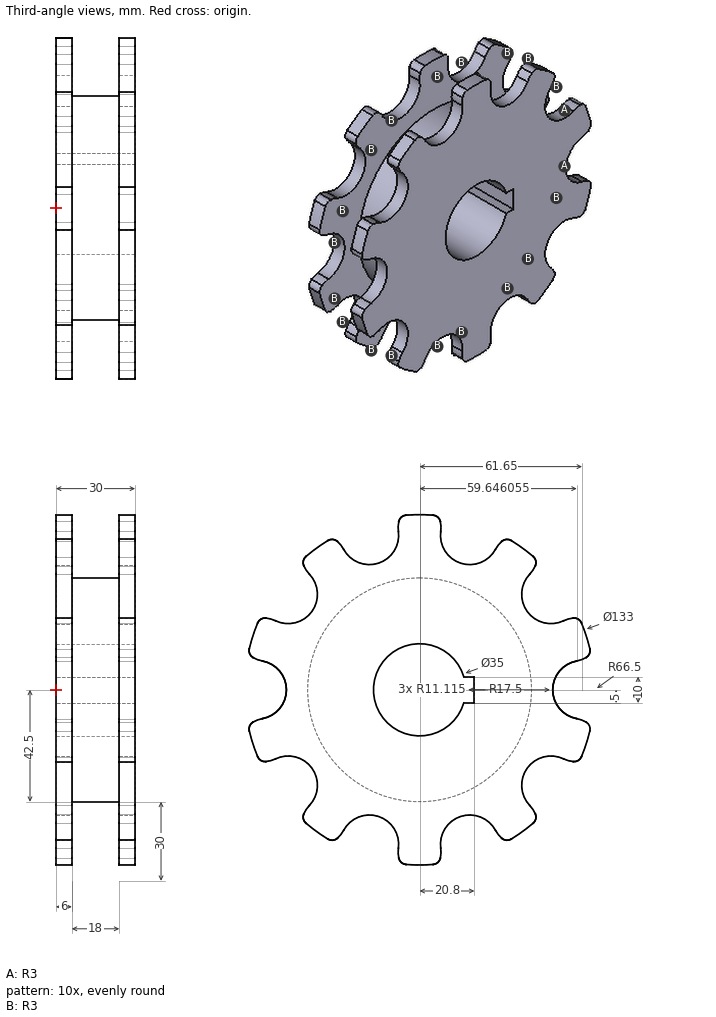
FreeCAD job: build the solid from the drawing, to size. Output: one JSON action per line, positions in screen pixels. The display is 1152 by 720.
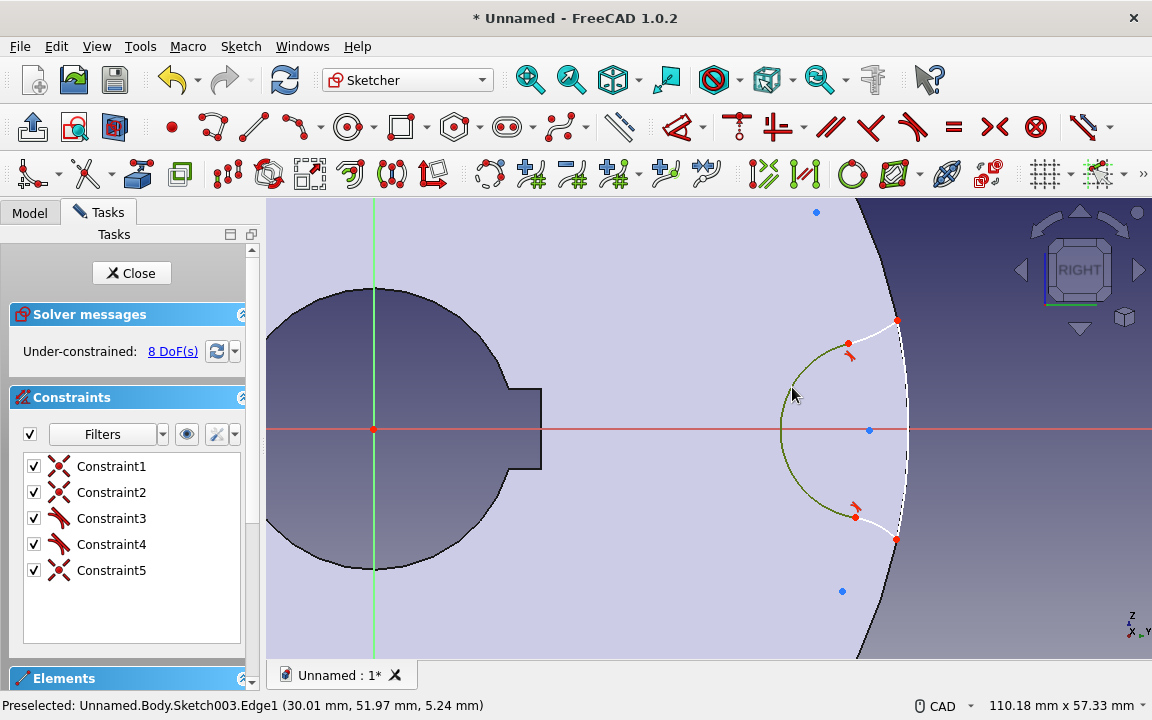
{"action": "left_click", "coordinate": [886, 530]}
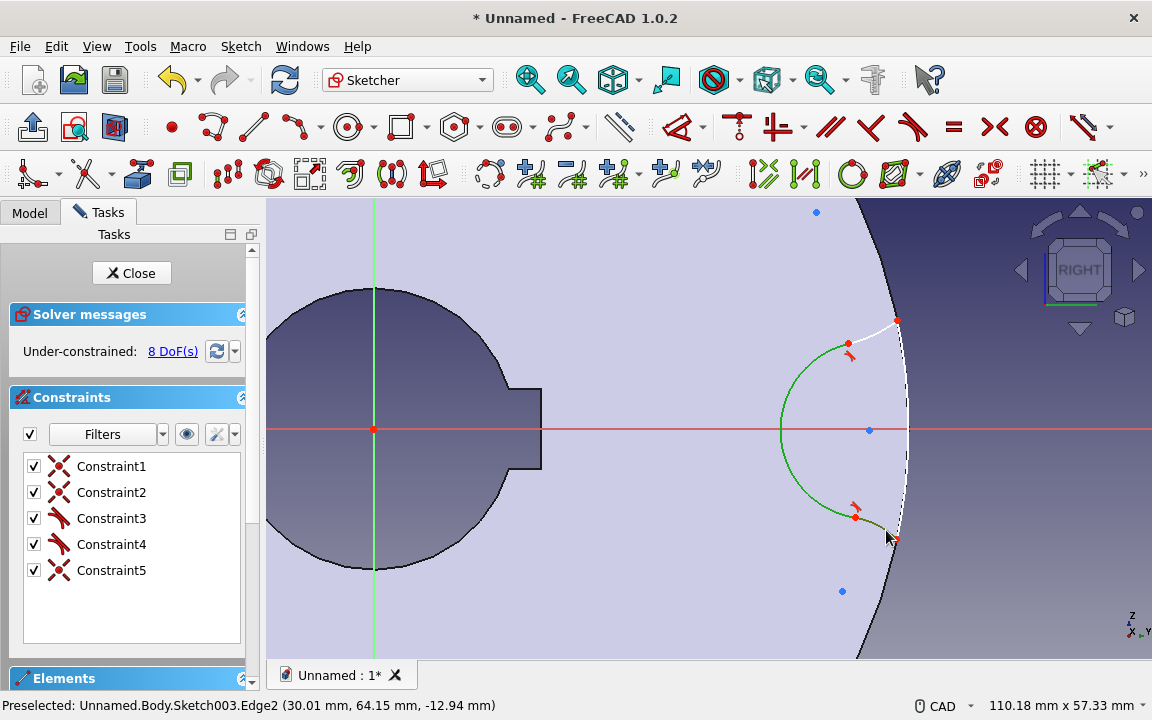
{"action": "left_click", "coordinate": [864, 339]}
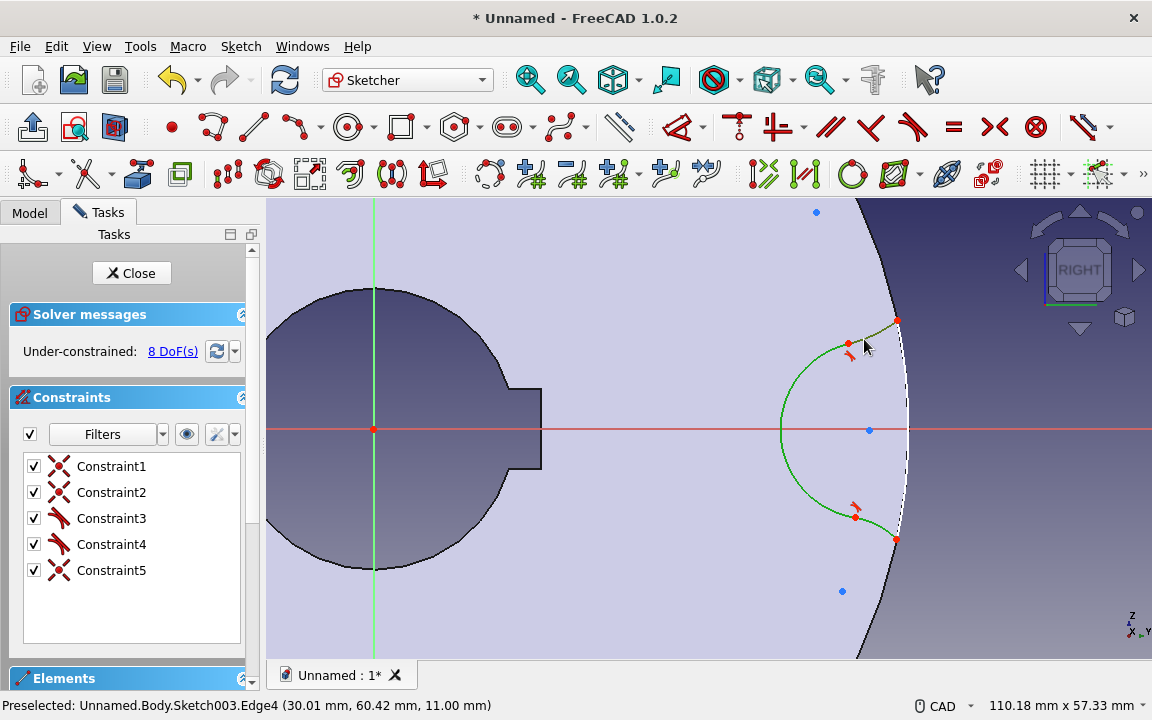
{"action": "left_click", "coordinate": [954, 128]}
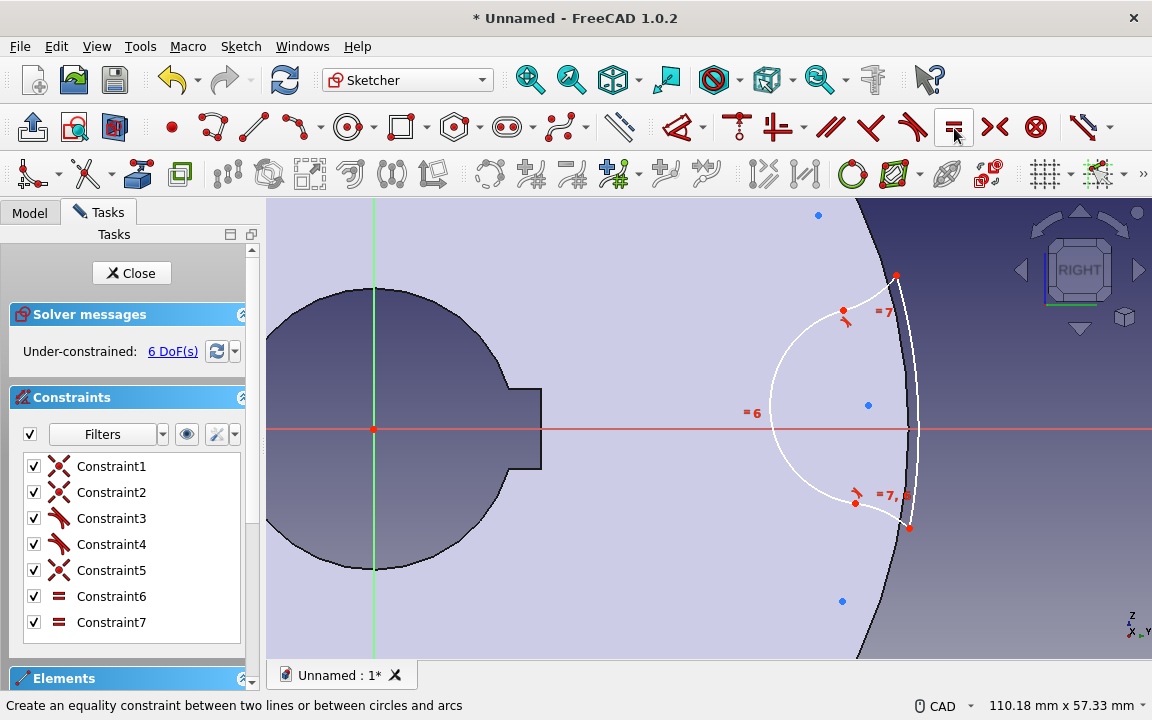
{"action": "left_click", "coordinate": [869, 406]}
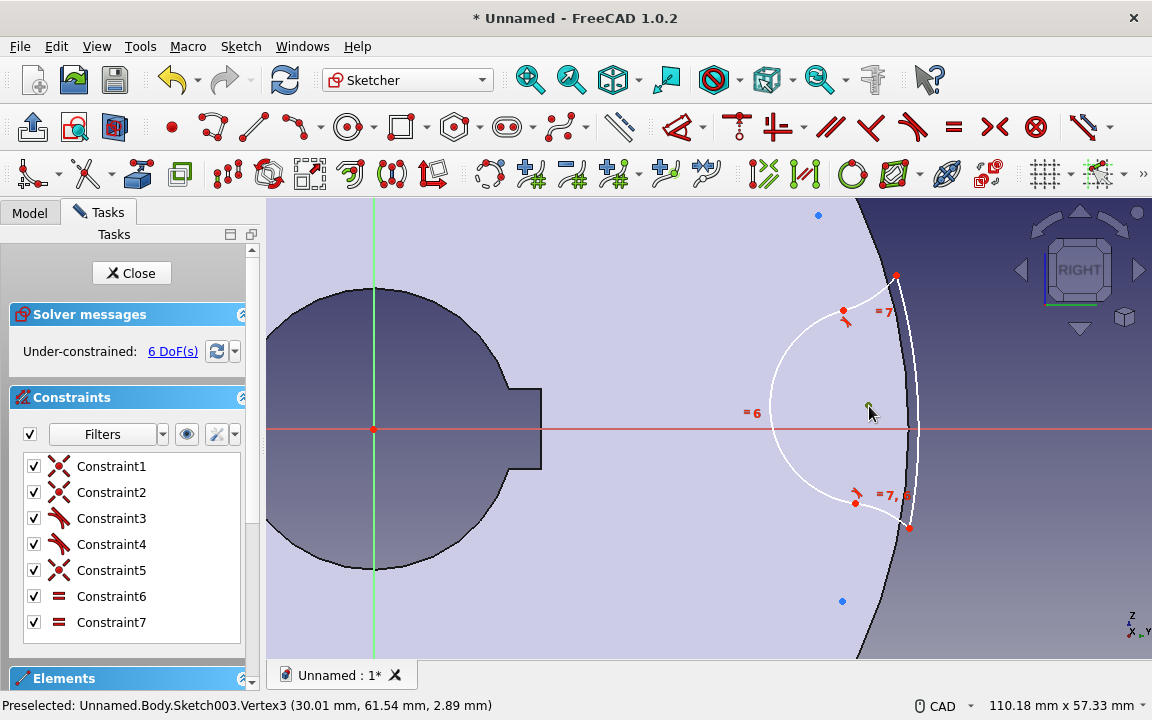
{"action": "left_click", "coordinate": [344, 429]}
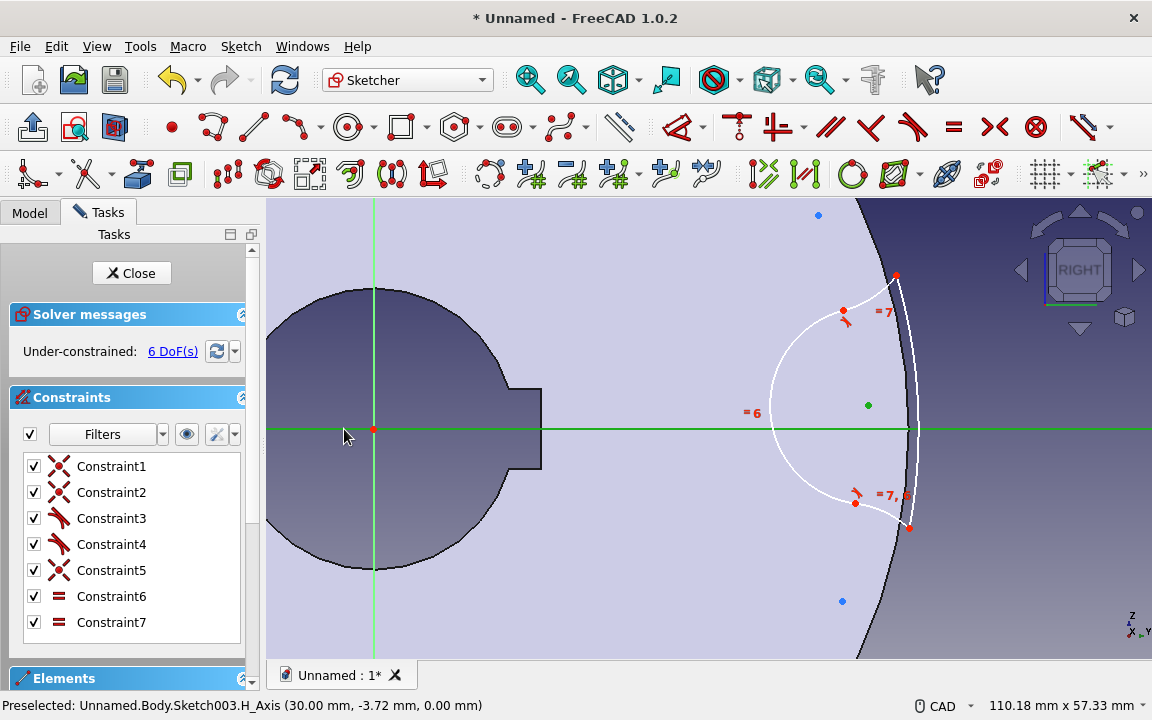
{"action": "left_click", "coordinate": [737, 128]}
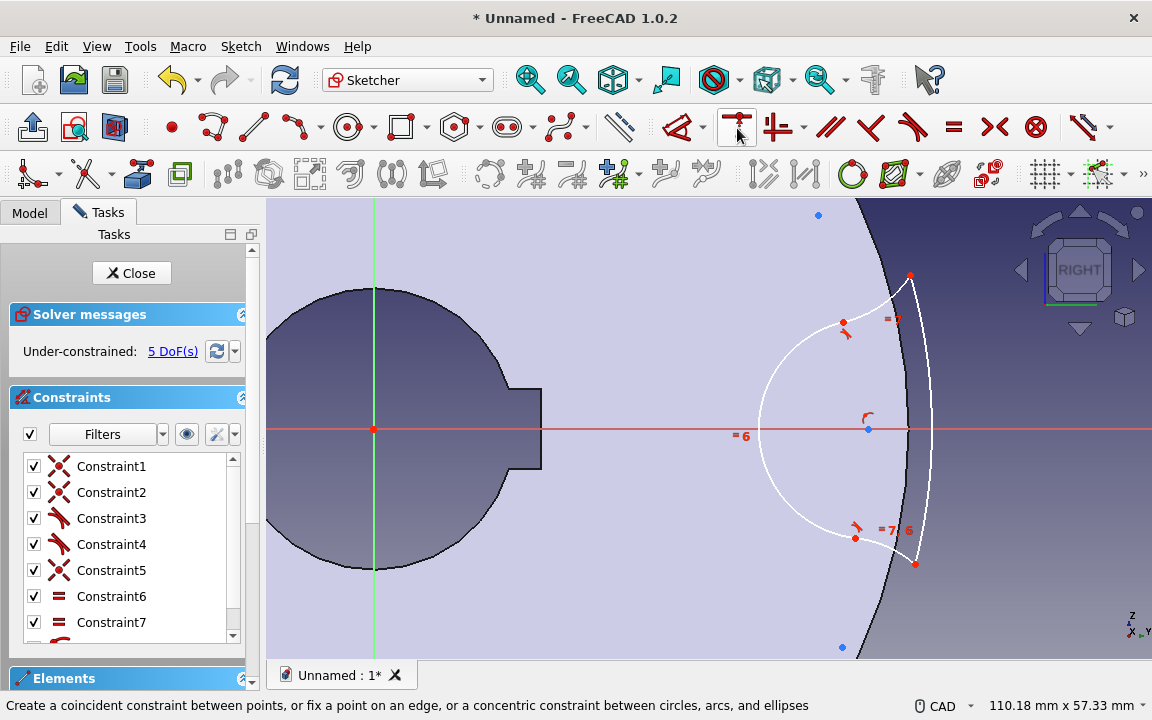
{"action": "left_click", "coordinate": [676, 128]}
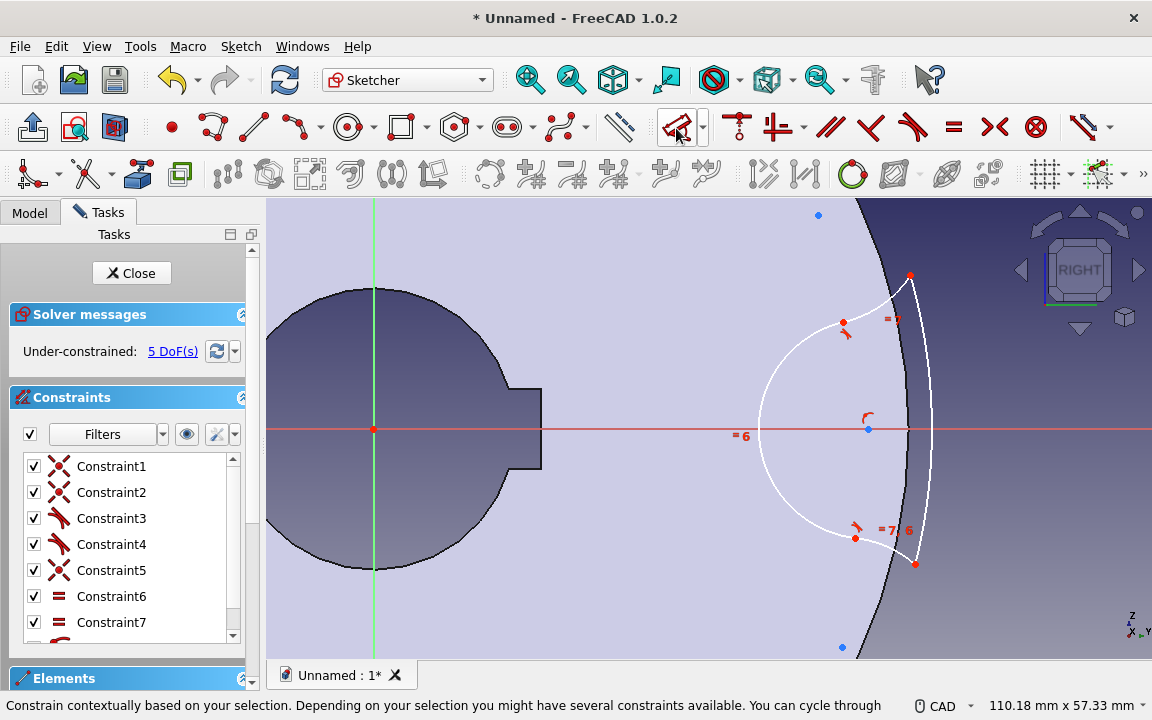
{"action": "left_click", "coordinate": [772, 376]}
{"action": "left_click", "coordinate": [744, 361]}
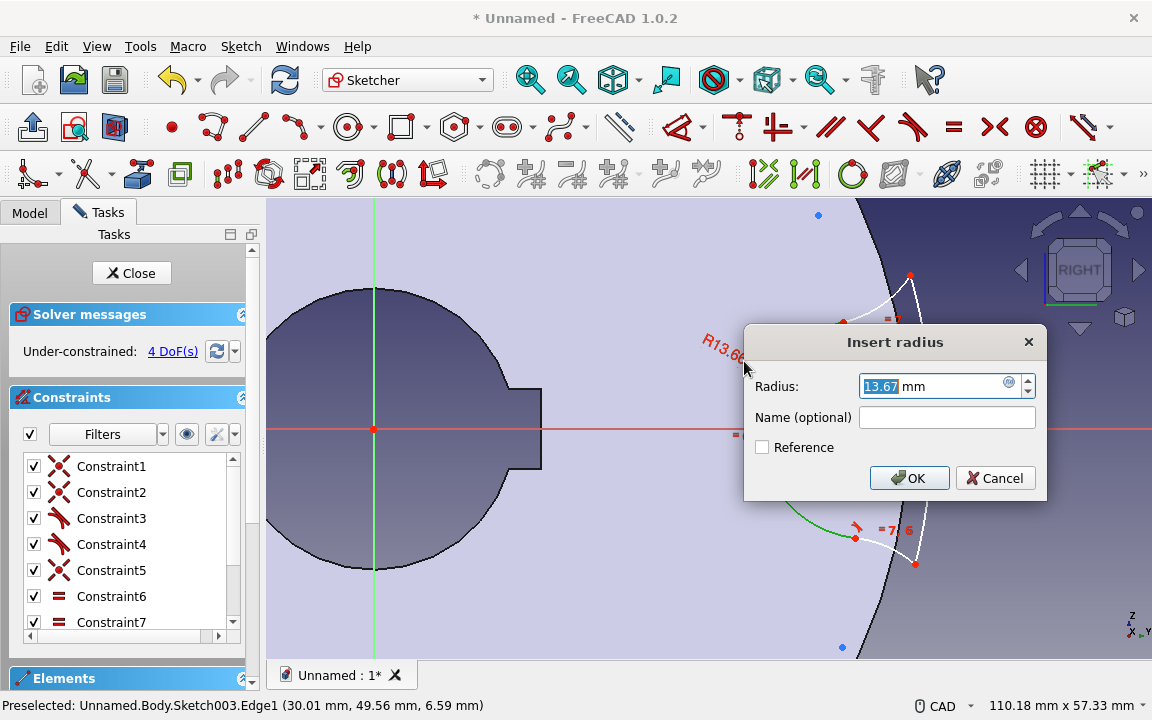
{"action": "type", "text": "11.115"}
{"action": "key", "text": "Return"}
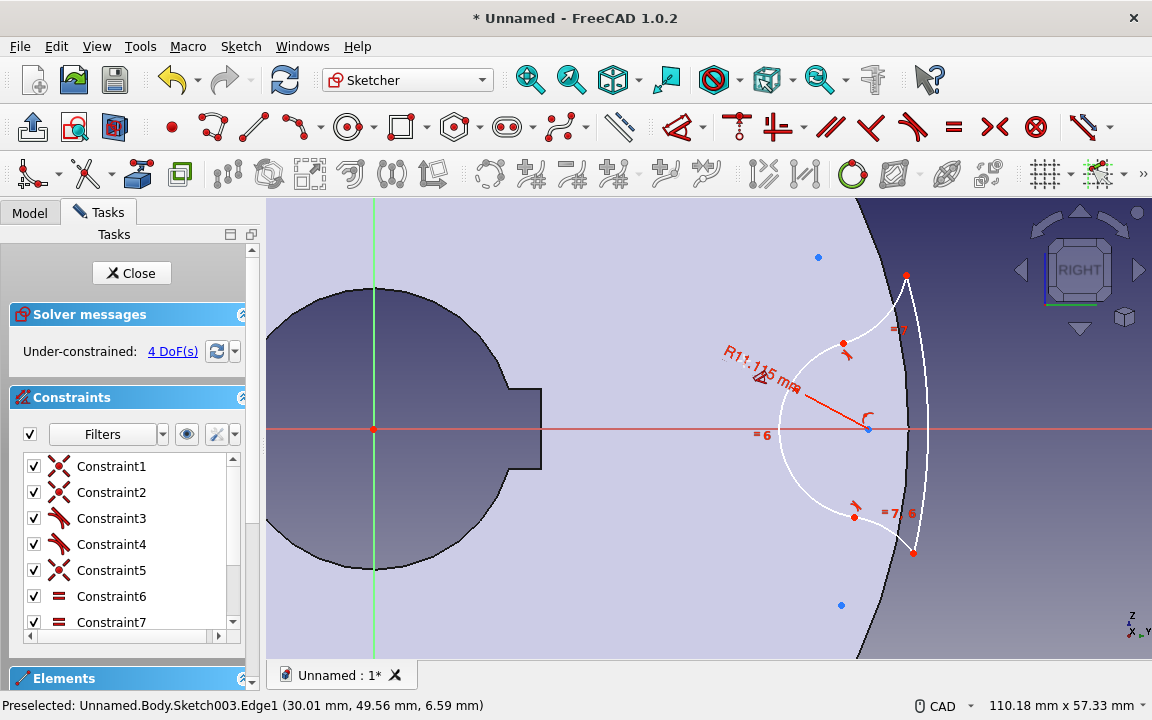
{"action": "left_click", "coordinate": [927, 470]}
{"action": "left_click", "coordinate": [959, 472]}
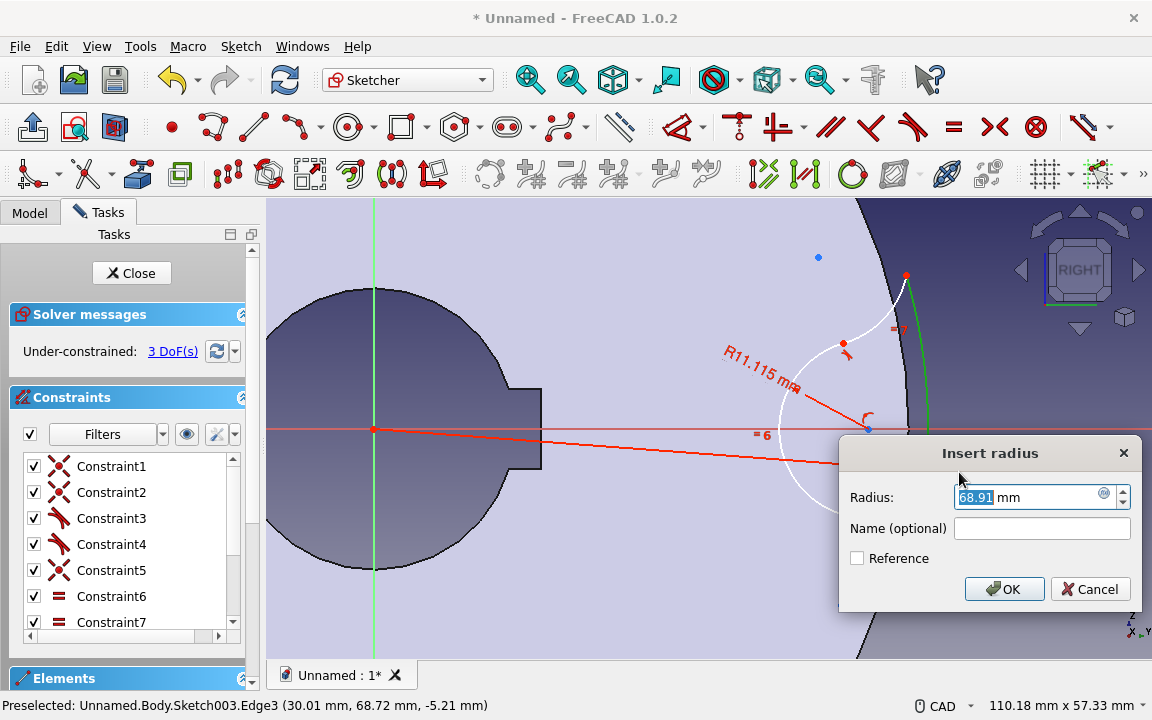
{"action": "type", "text": "66.5"}
{"action": "key", "text": "Return"}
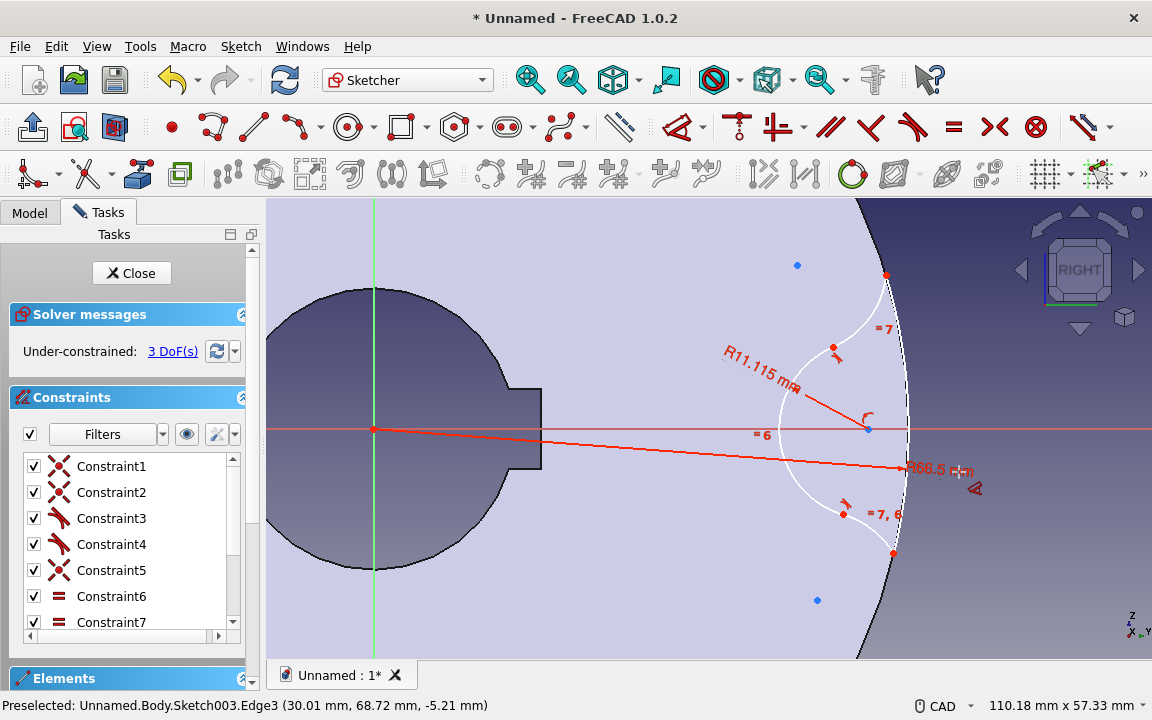
{"action": "left_click", "coordinate": [869, 429]}
{"action": "left_click", "coordinate": [621, 463]}